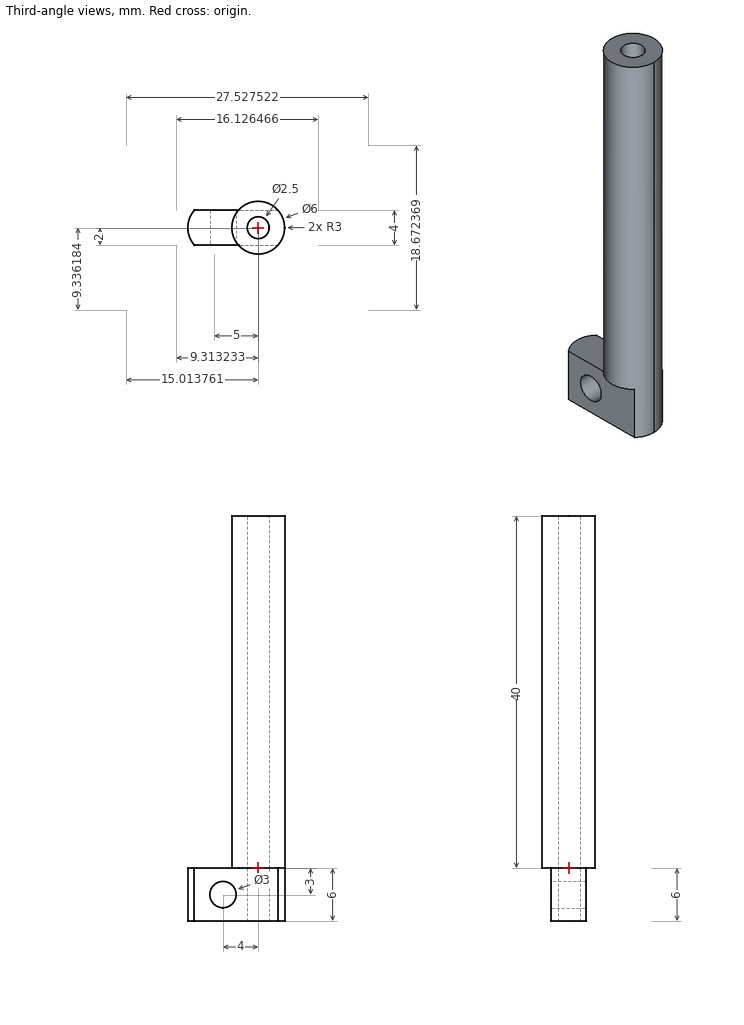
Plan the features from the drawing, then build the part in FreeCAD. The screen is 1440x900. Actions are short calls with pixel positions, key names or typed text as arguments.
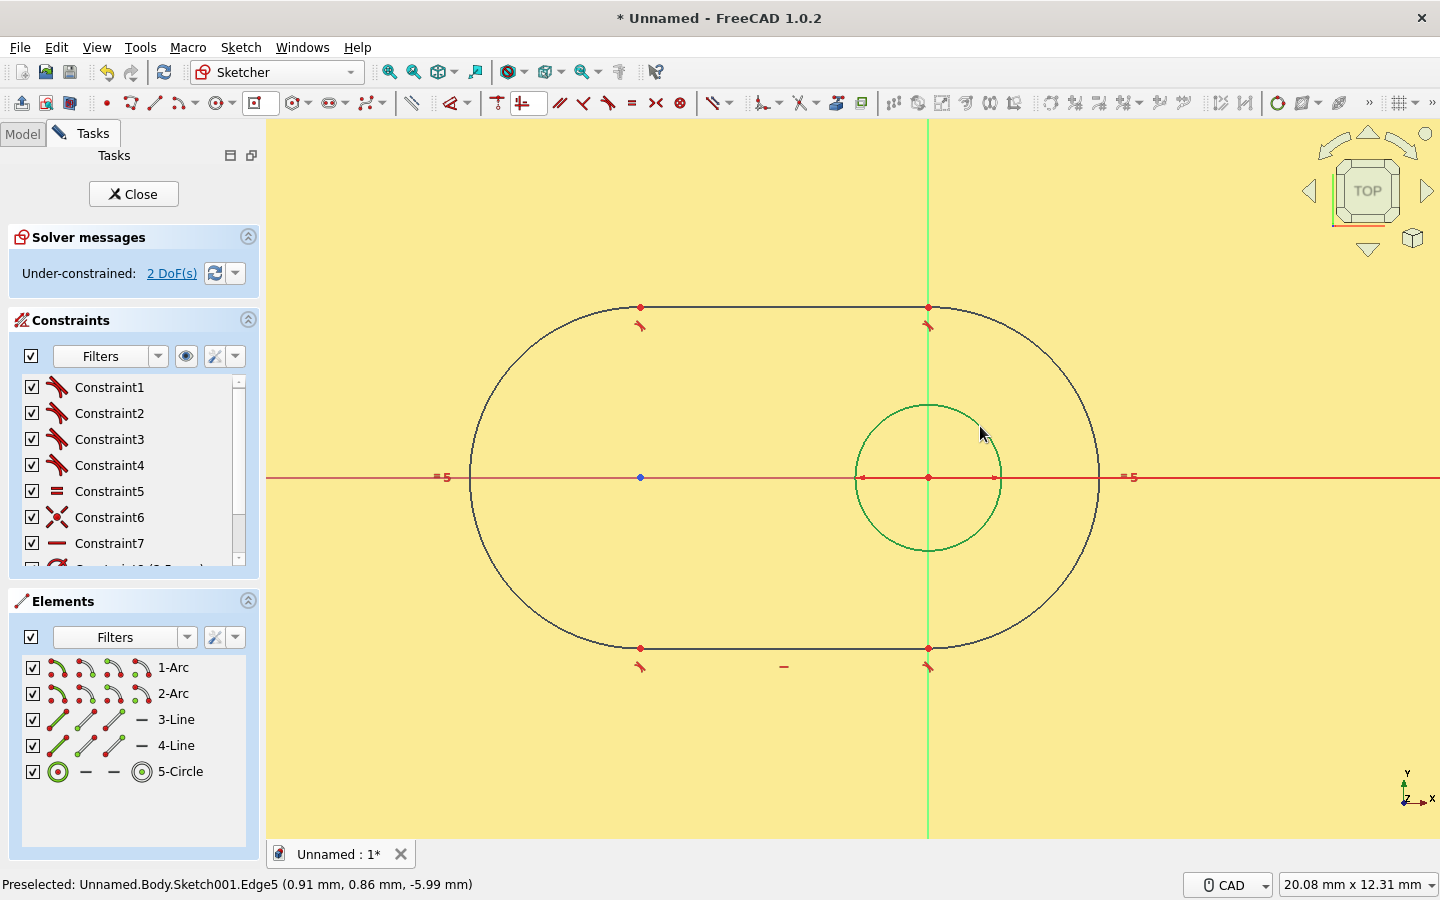
key(d)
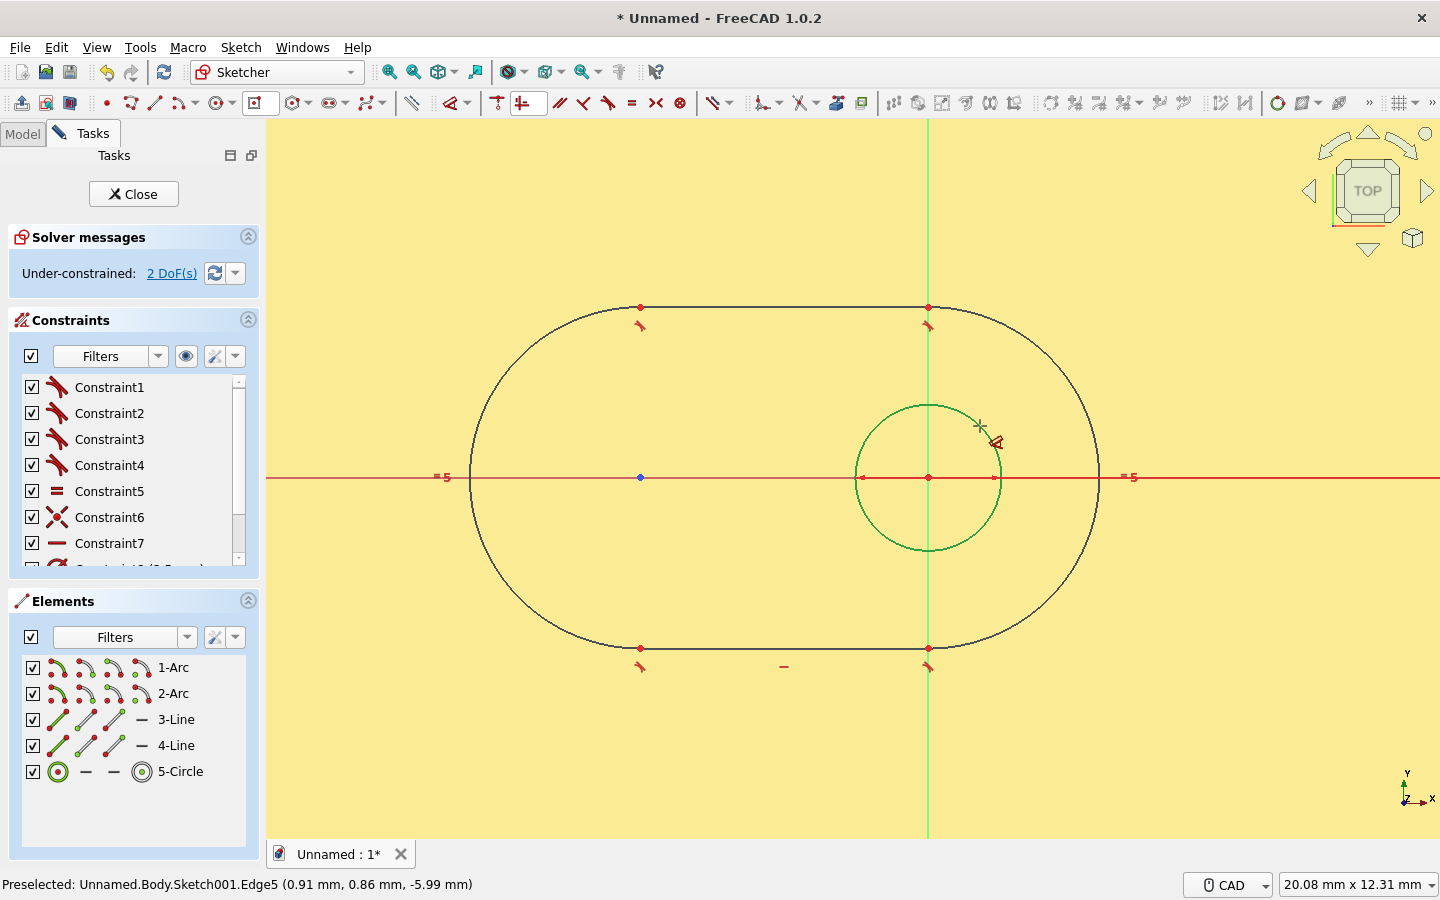
click(1067, 578)
click(1093, 597)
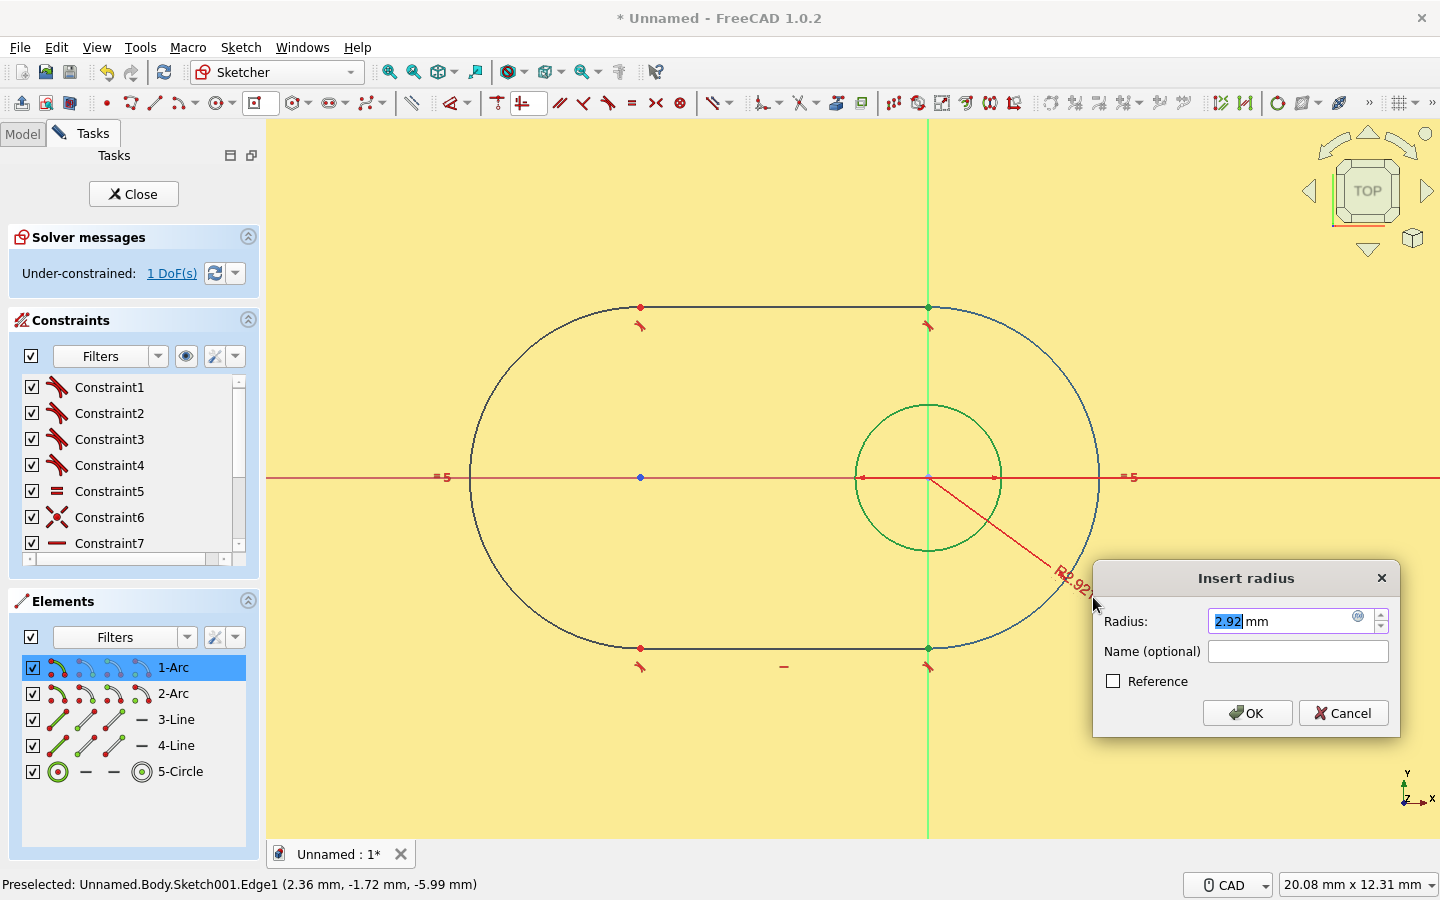
text(3)
key(Return)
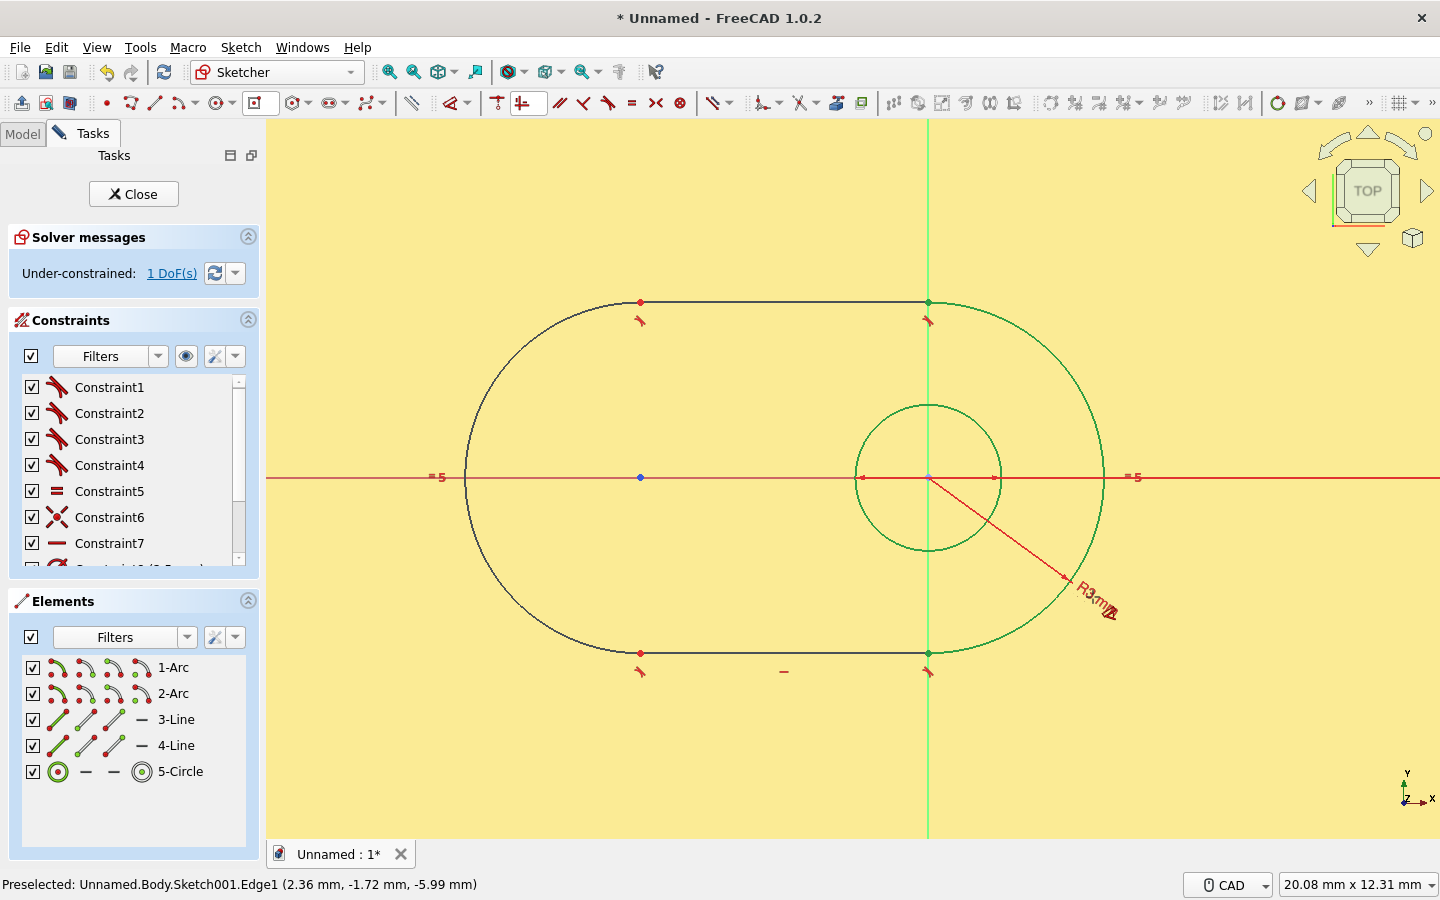
click(842, 653)
click(785, 687)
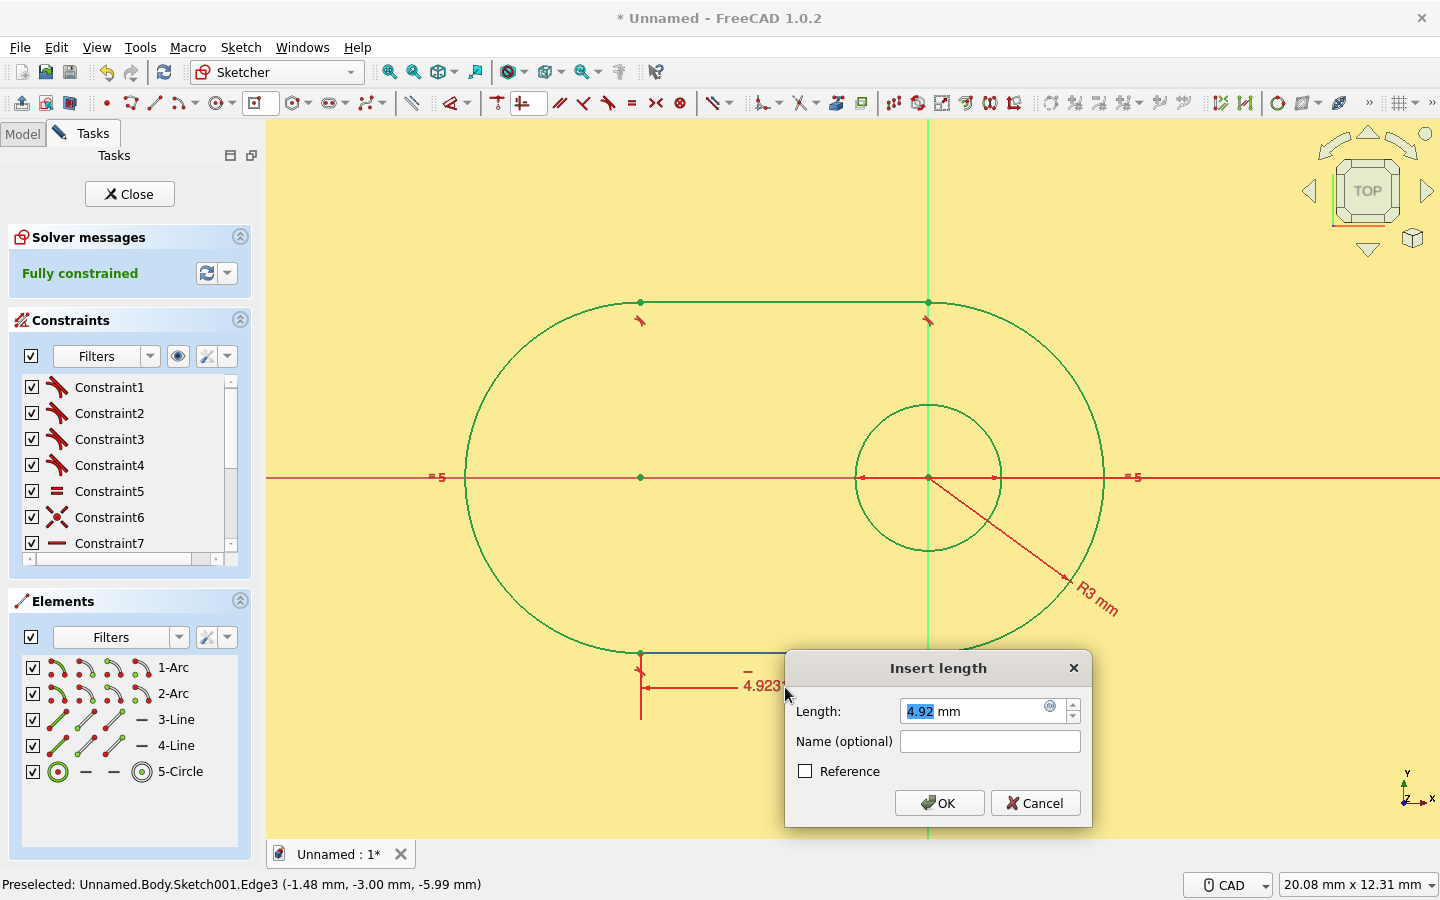
text(5)
key(Return)
key(Escape)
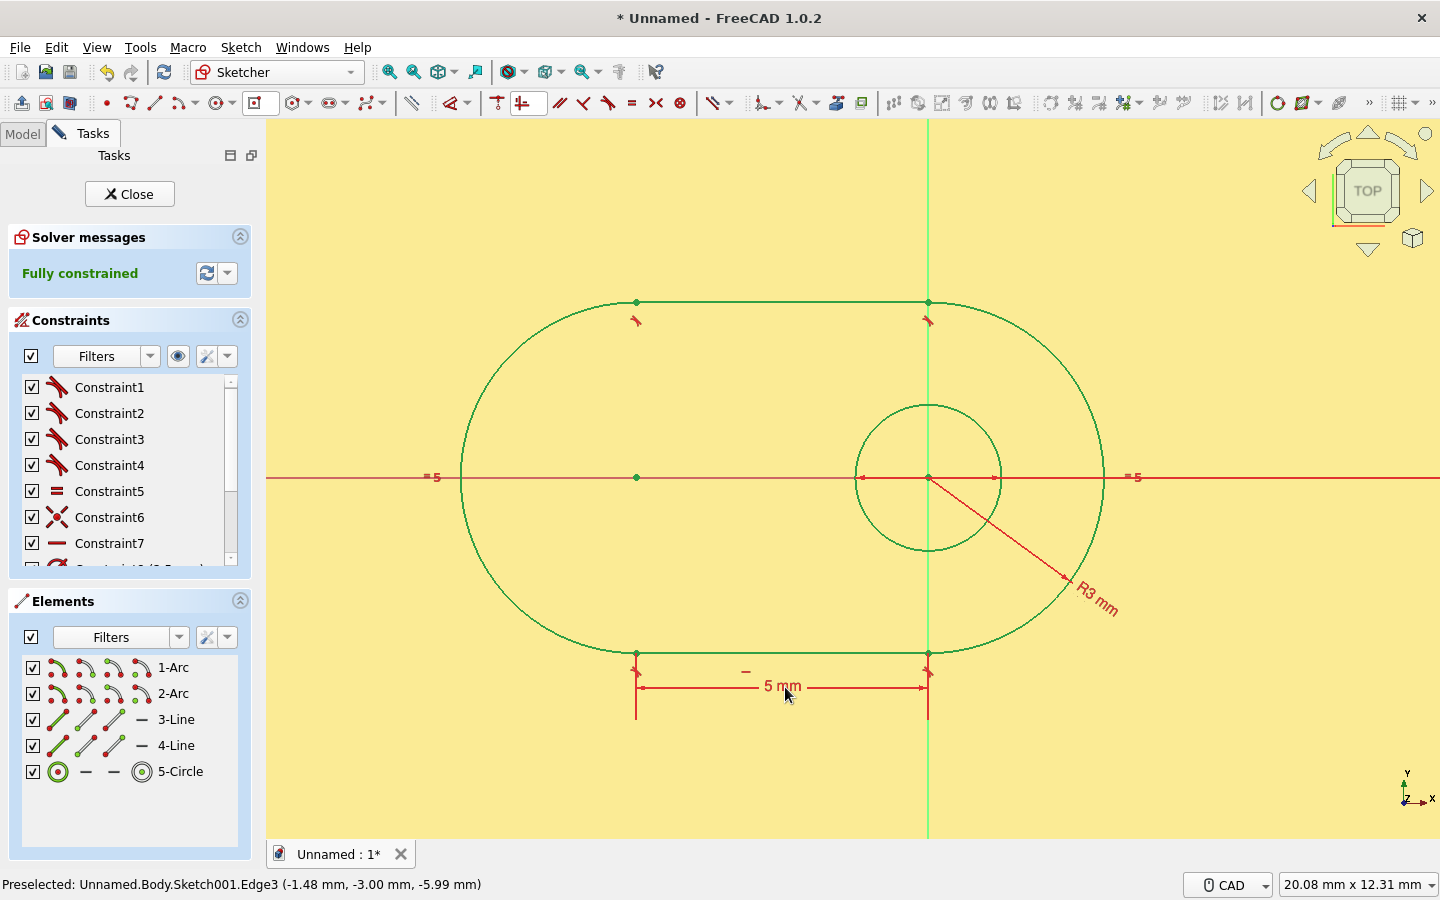
click(130, 194)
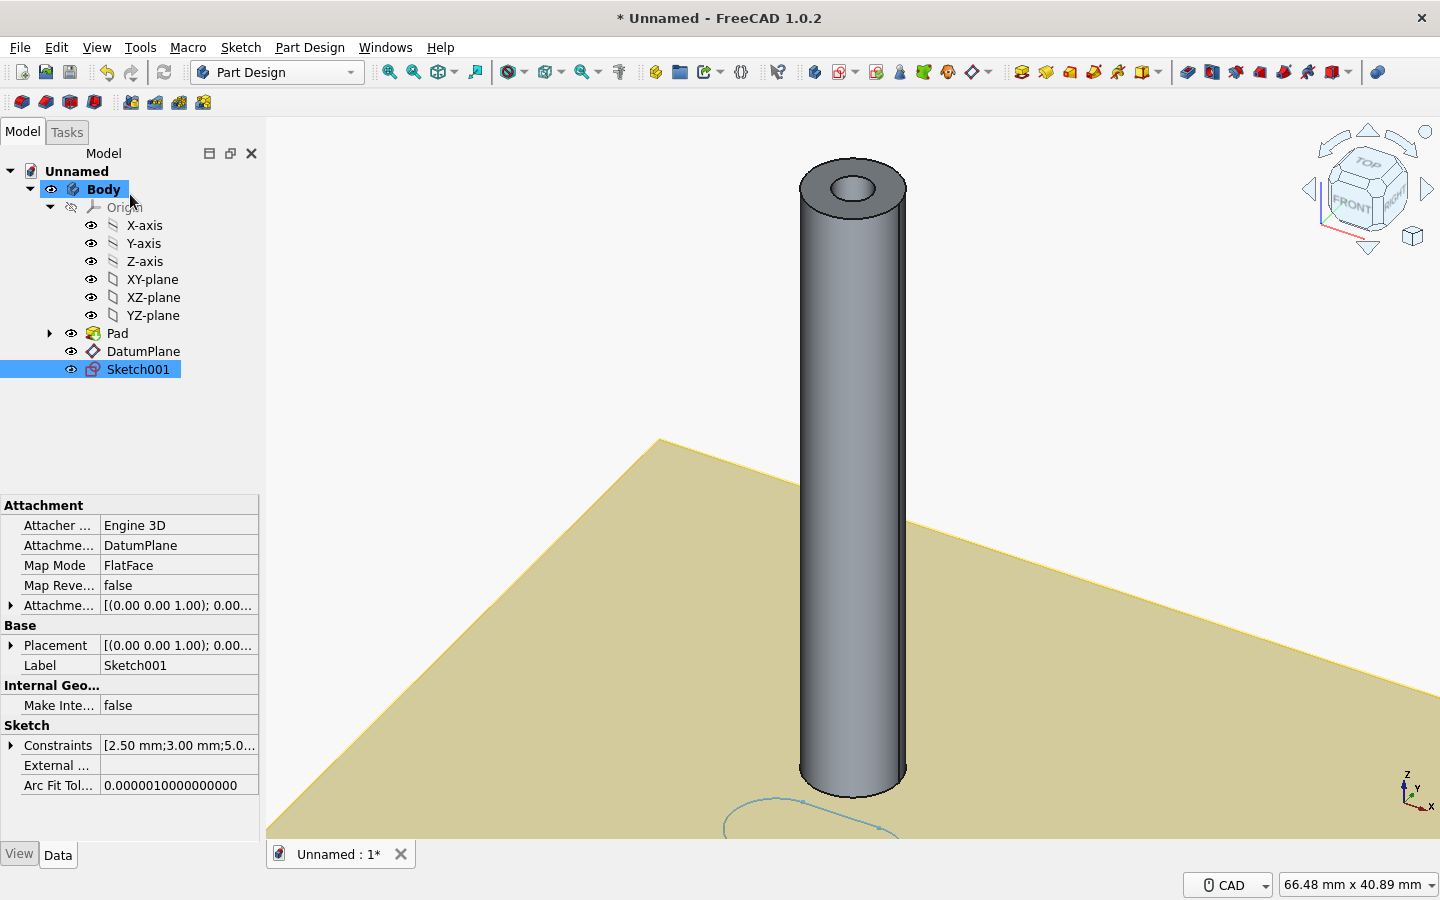
click(1022, 72)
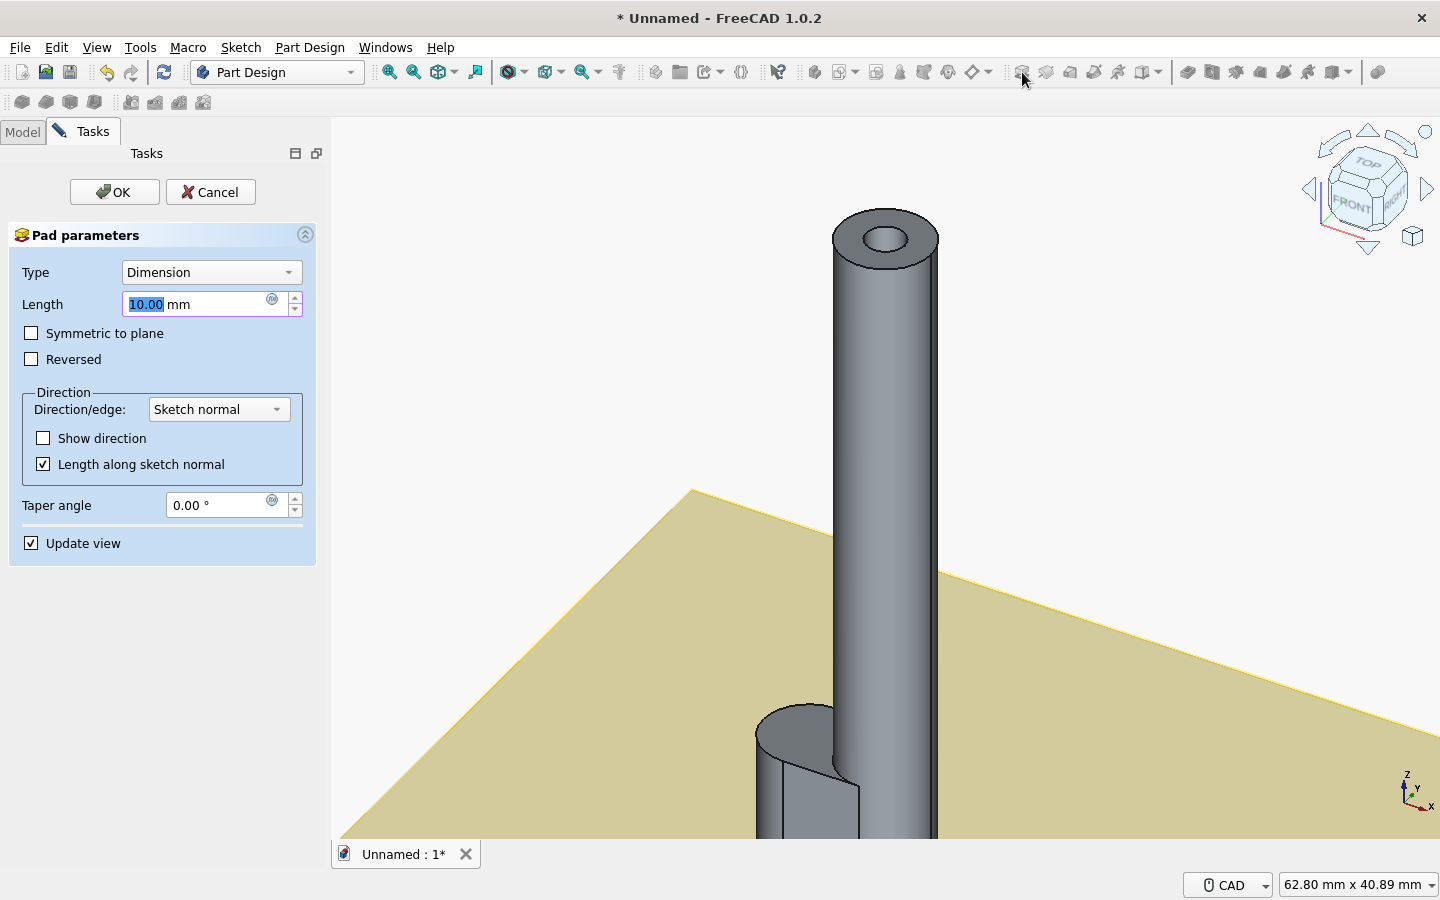
text(6)
key(Tab)